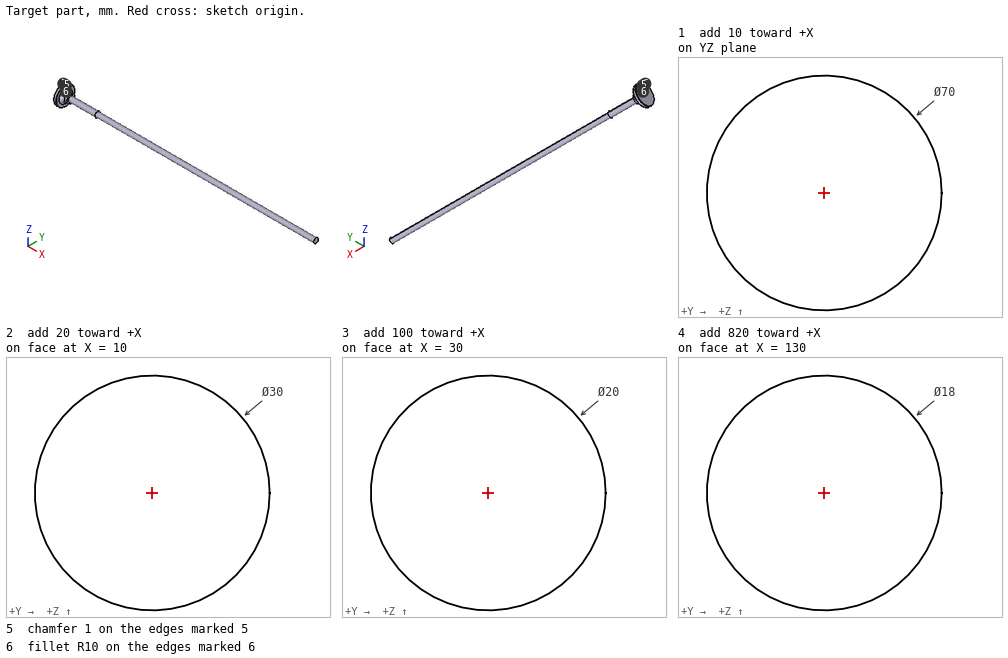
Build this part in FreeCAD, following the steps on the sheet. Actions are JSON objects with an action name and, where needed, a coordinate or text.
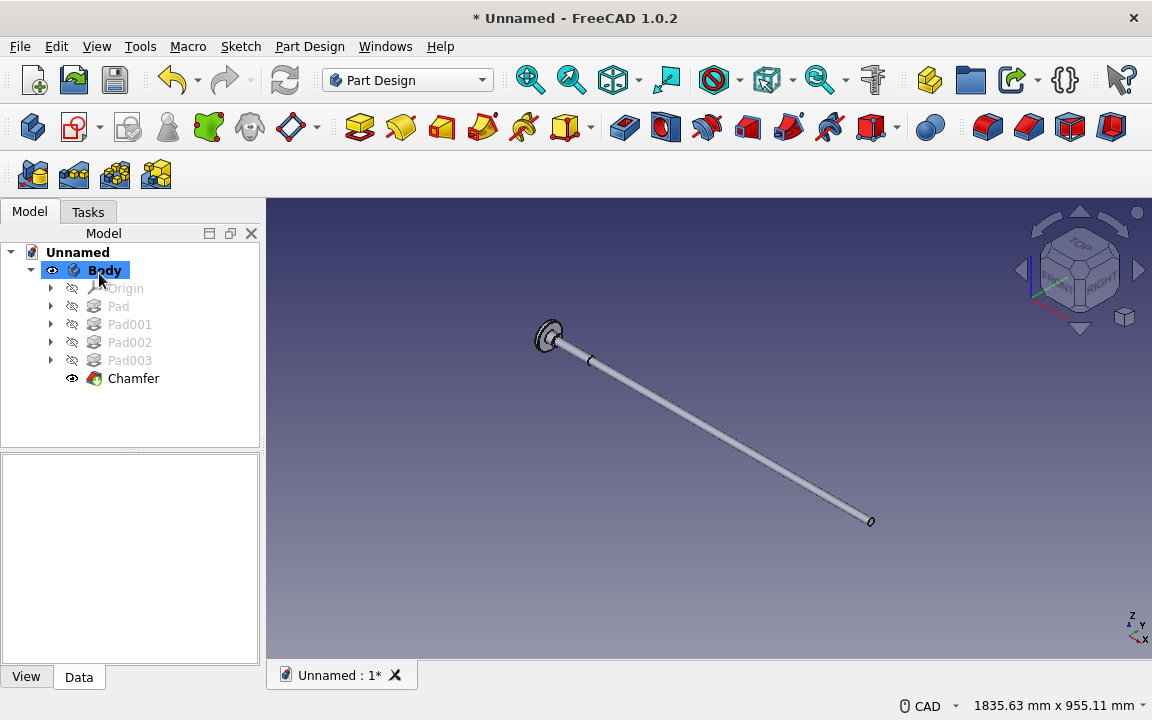
{"action": "left_click", "coordinate": [546, 342]}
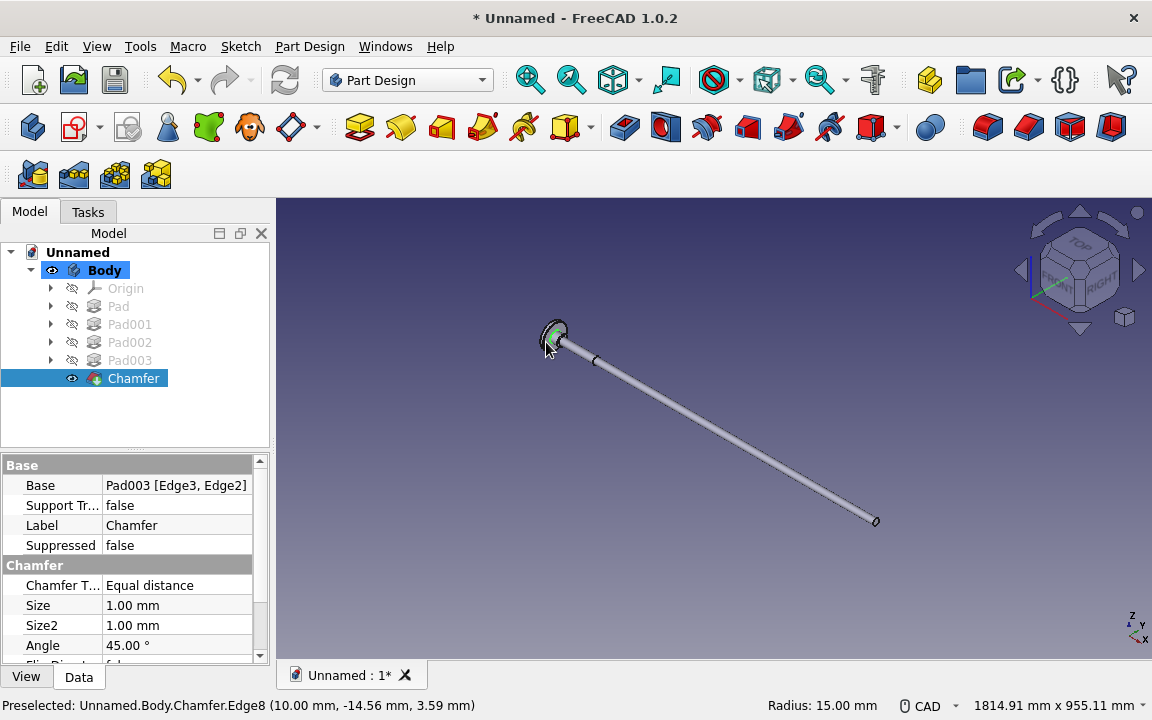
{"action": "left_click", "coordinate": [988, 128]}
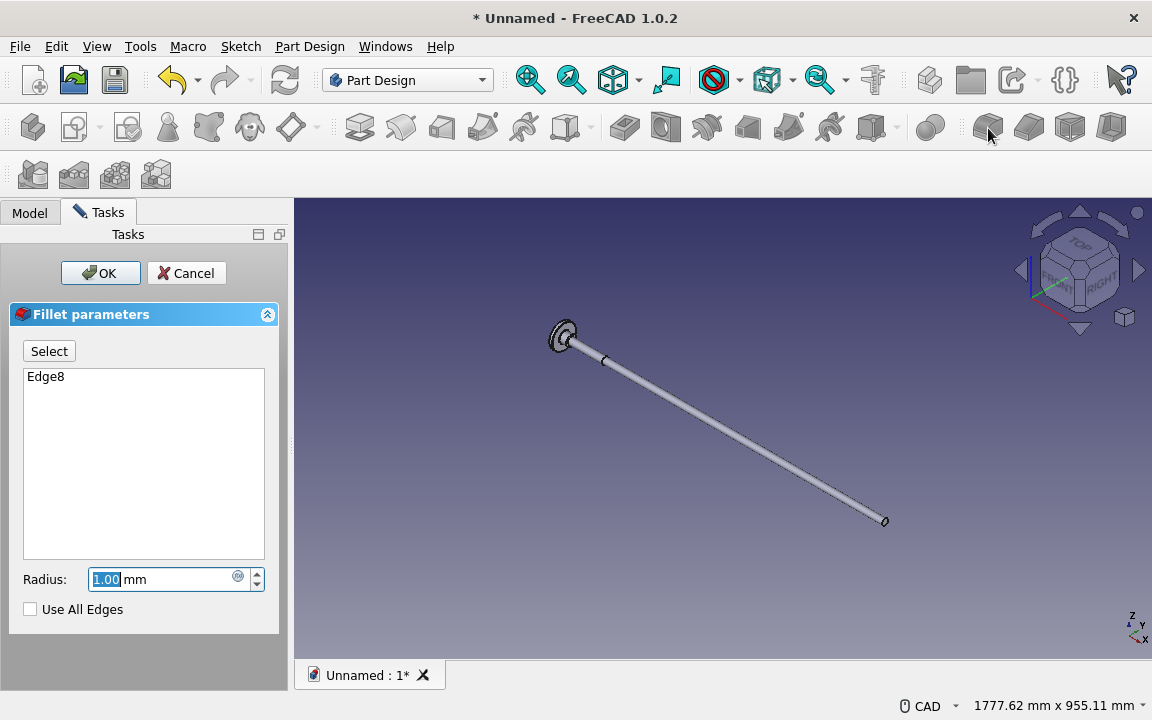
{"action": "type", "text": "10"}
{"action": "key", "text": "Tab"}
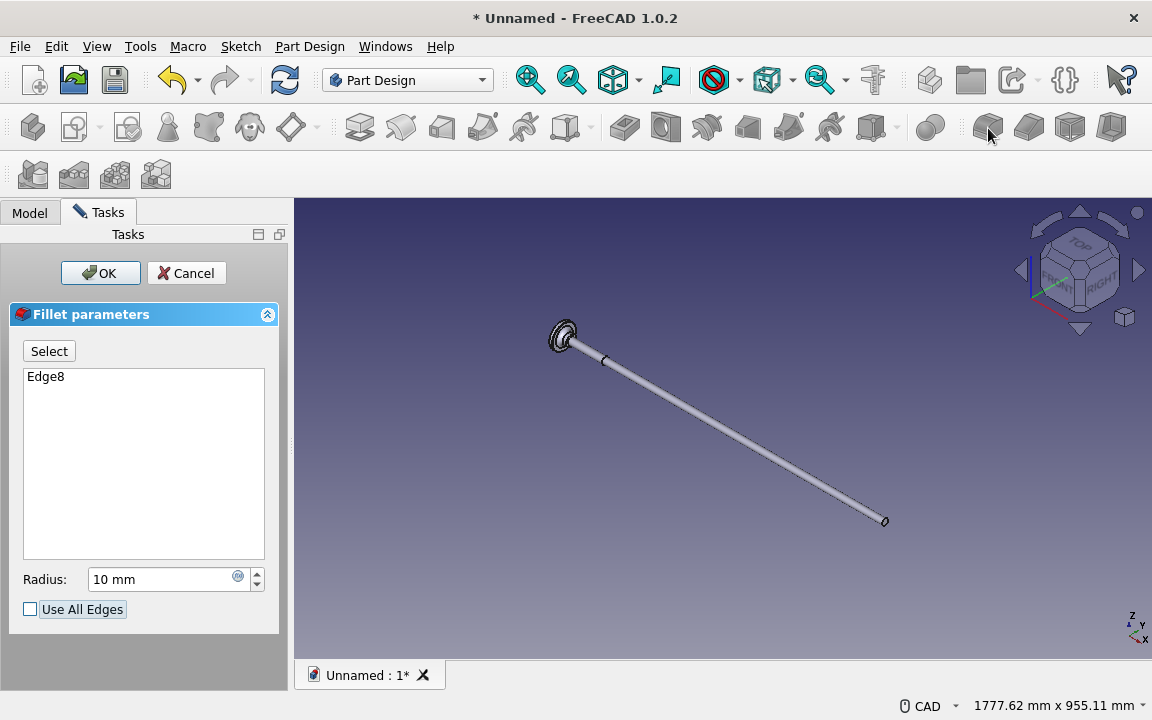
{"action": "left_click", "coordinate": [101, 273]}